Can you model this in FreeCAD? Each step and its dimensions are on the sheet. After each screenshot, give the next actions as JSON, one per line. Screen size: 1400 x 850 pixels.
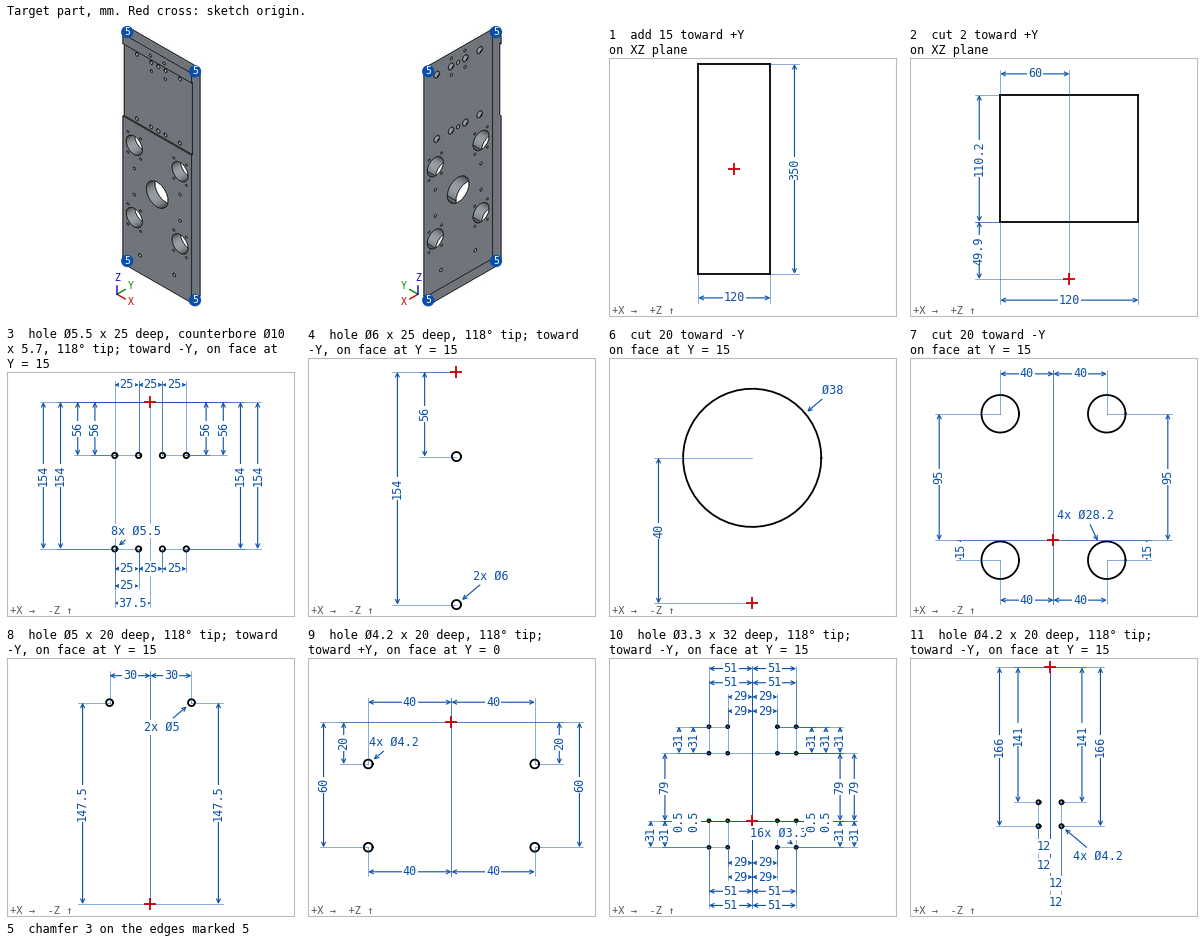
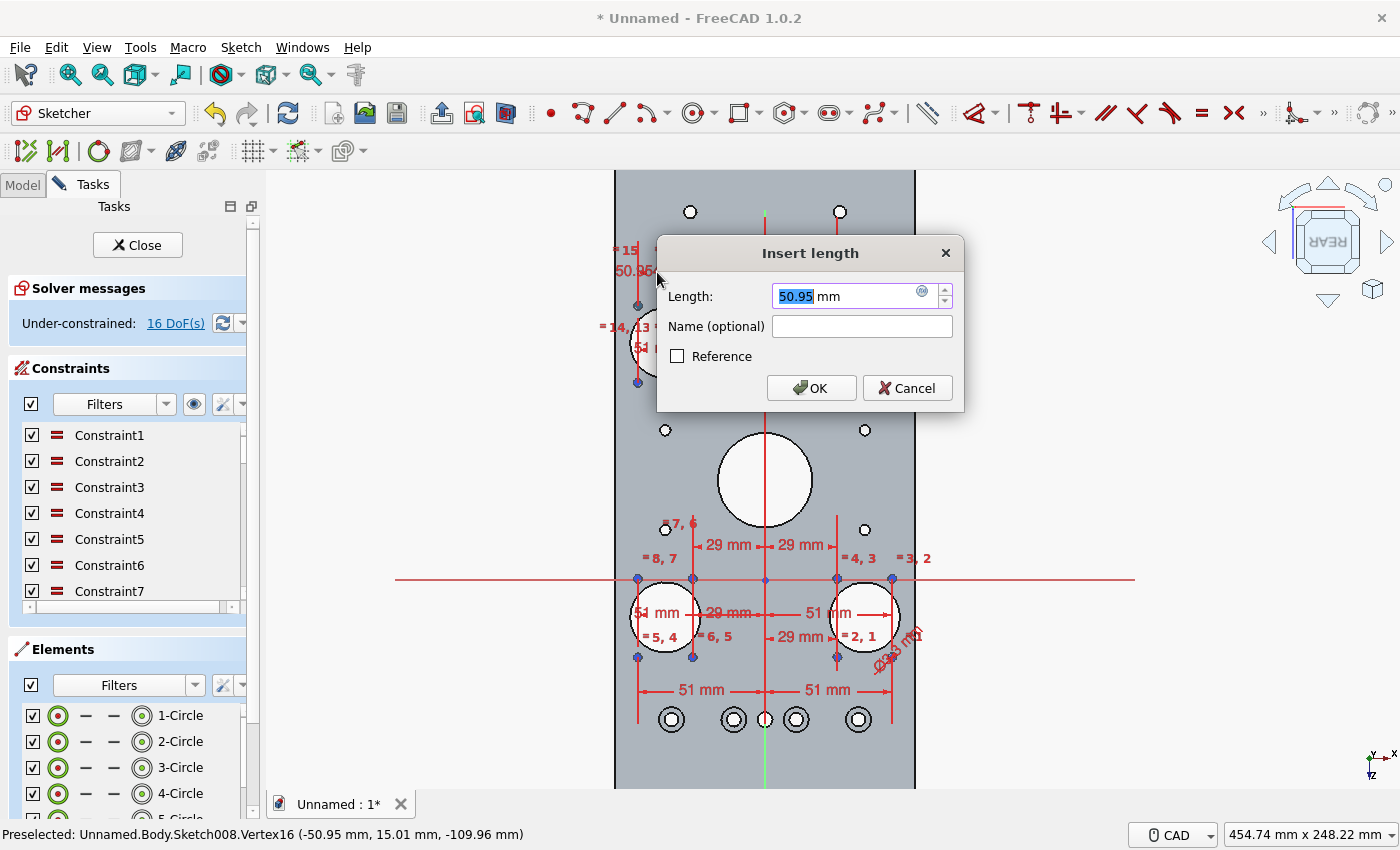
{"action": "type", "text": "51"}
{"action": "key", "text": "Return"}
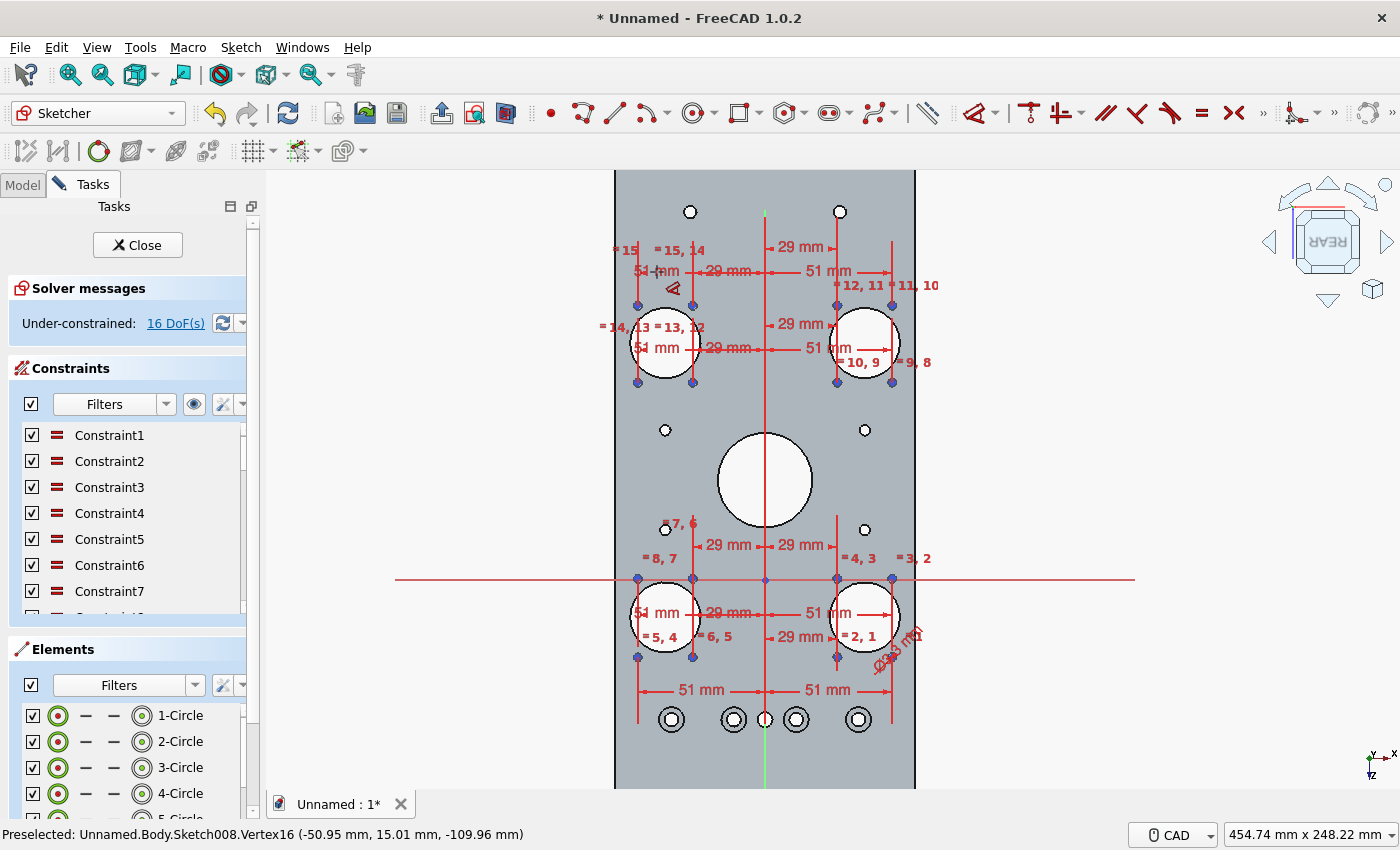
{"action": "scroll", "coordinate": [892, 579], "scroll_direction": "up", "scroll_amount": 18}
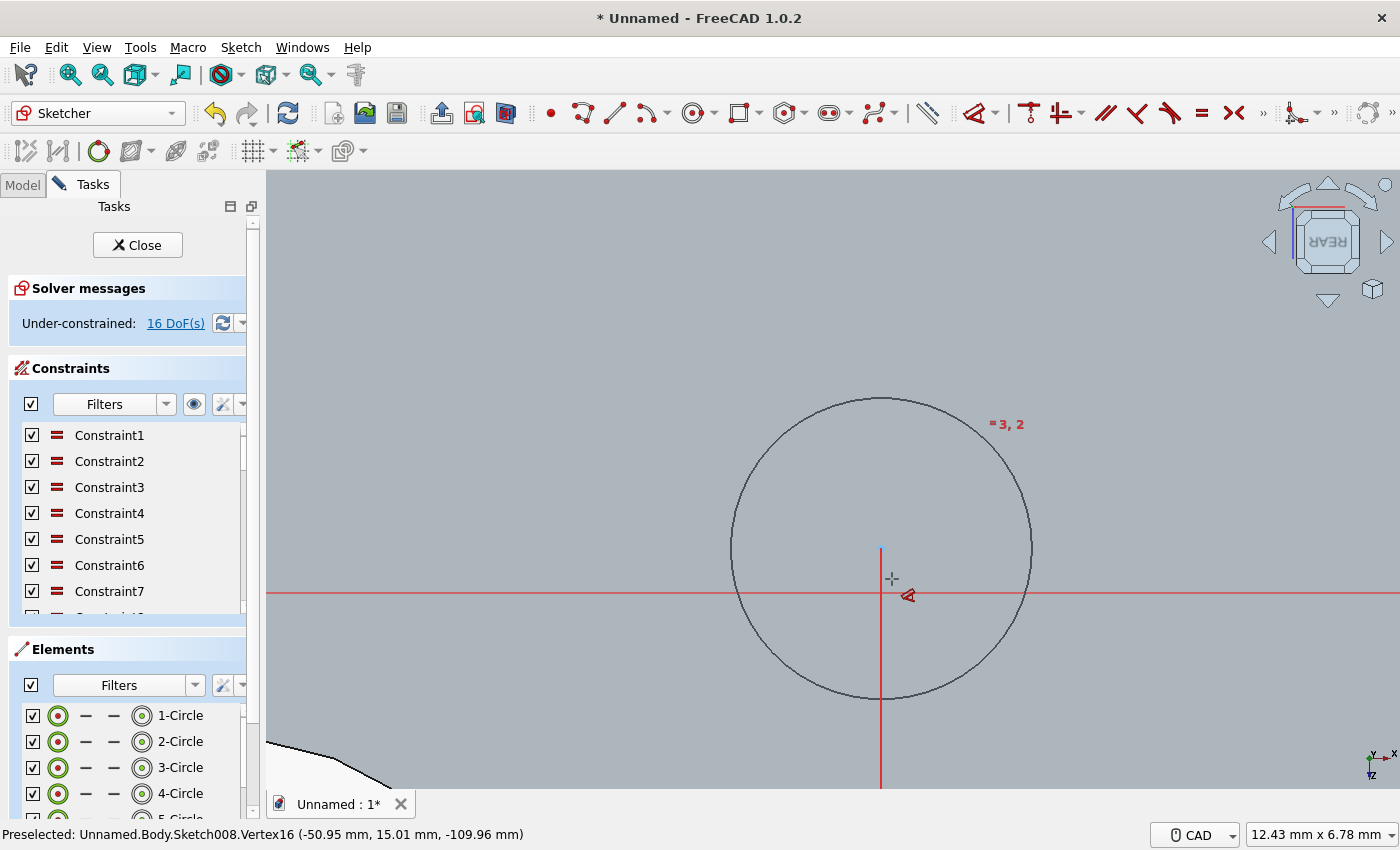
{"action": "left_click", "coordinate": [881, 549]}
{"action": "left_click", "coordinate": [915, 571]}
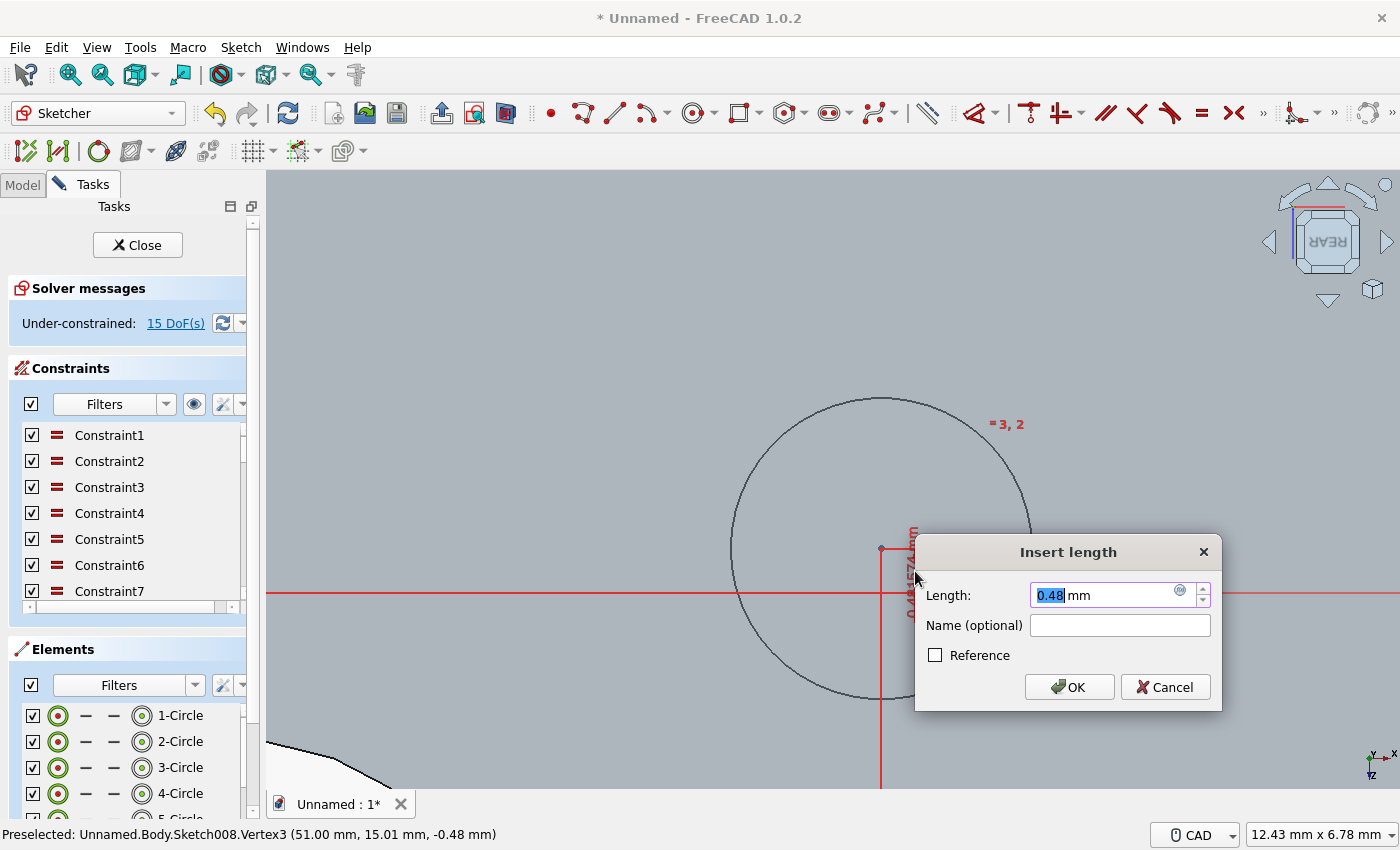
{"action": "type", "text": "0.5"}
{"action": "key", "text": "Return"}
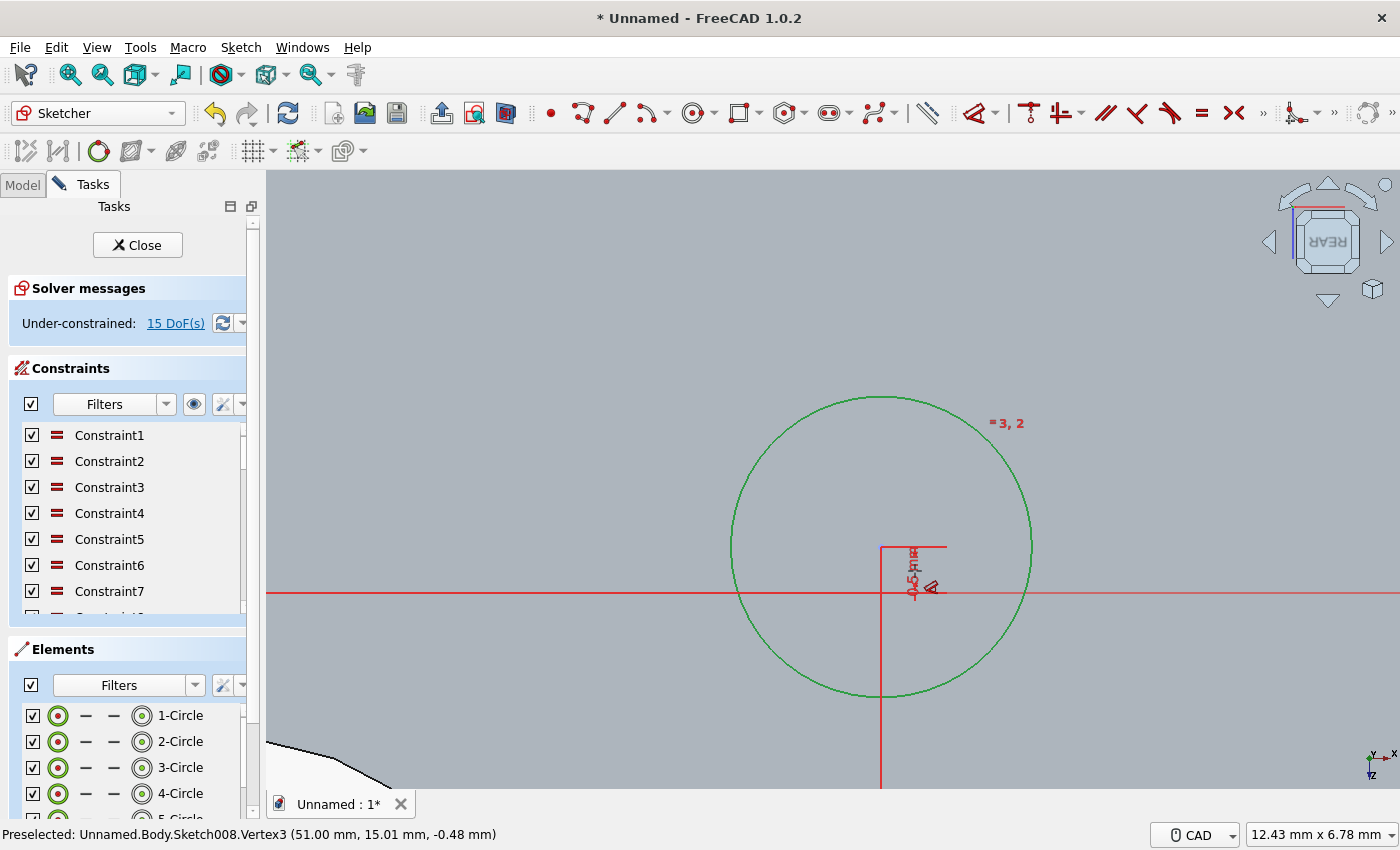
{"action": "scroll", "coordinate": [921, 602], "scroll_direction": "down", "scroll_amount": 17}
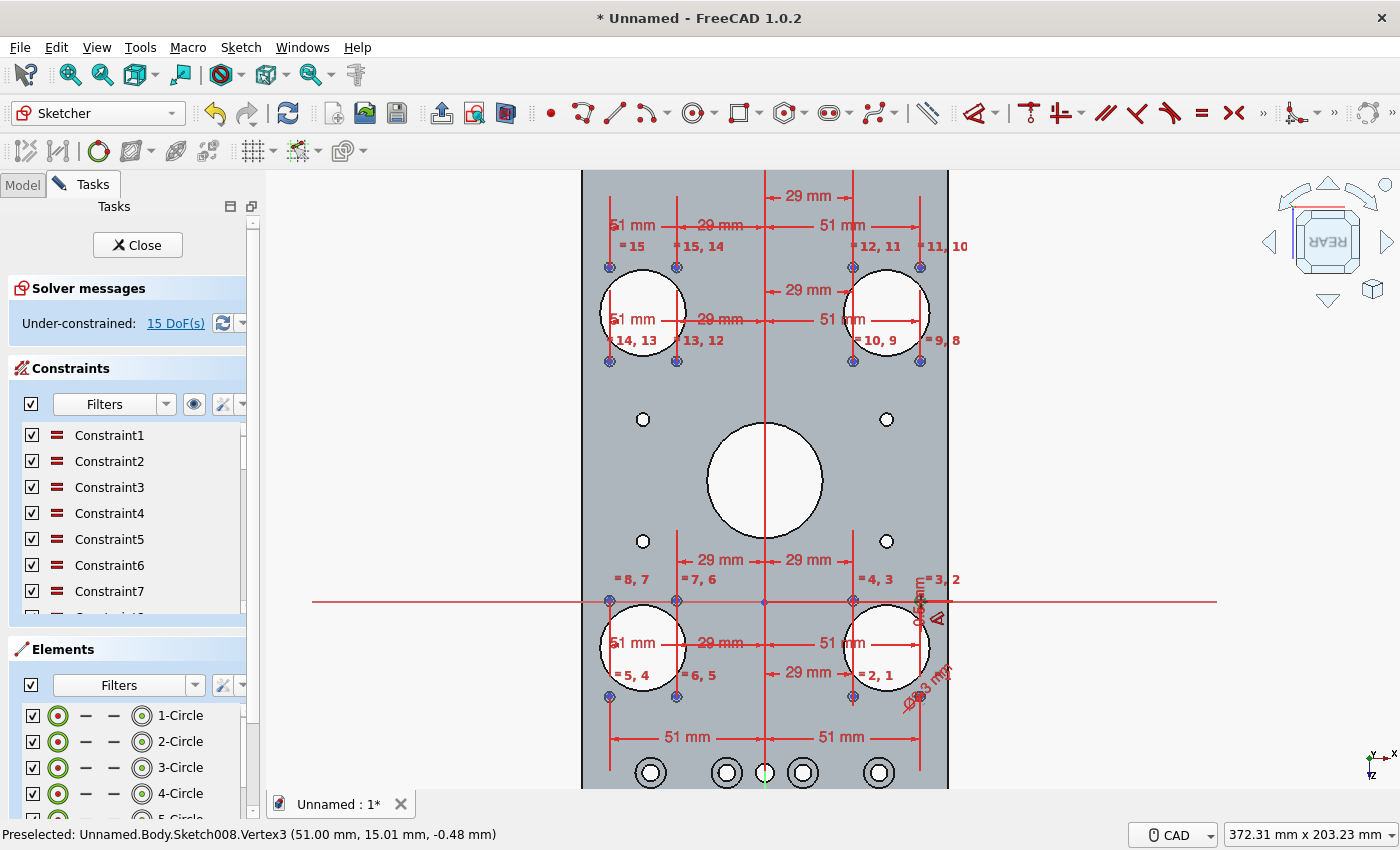
{"action": "scroll", "coordinate": [853, 601], "scroll_direction": "up", "scroll_amount": 17}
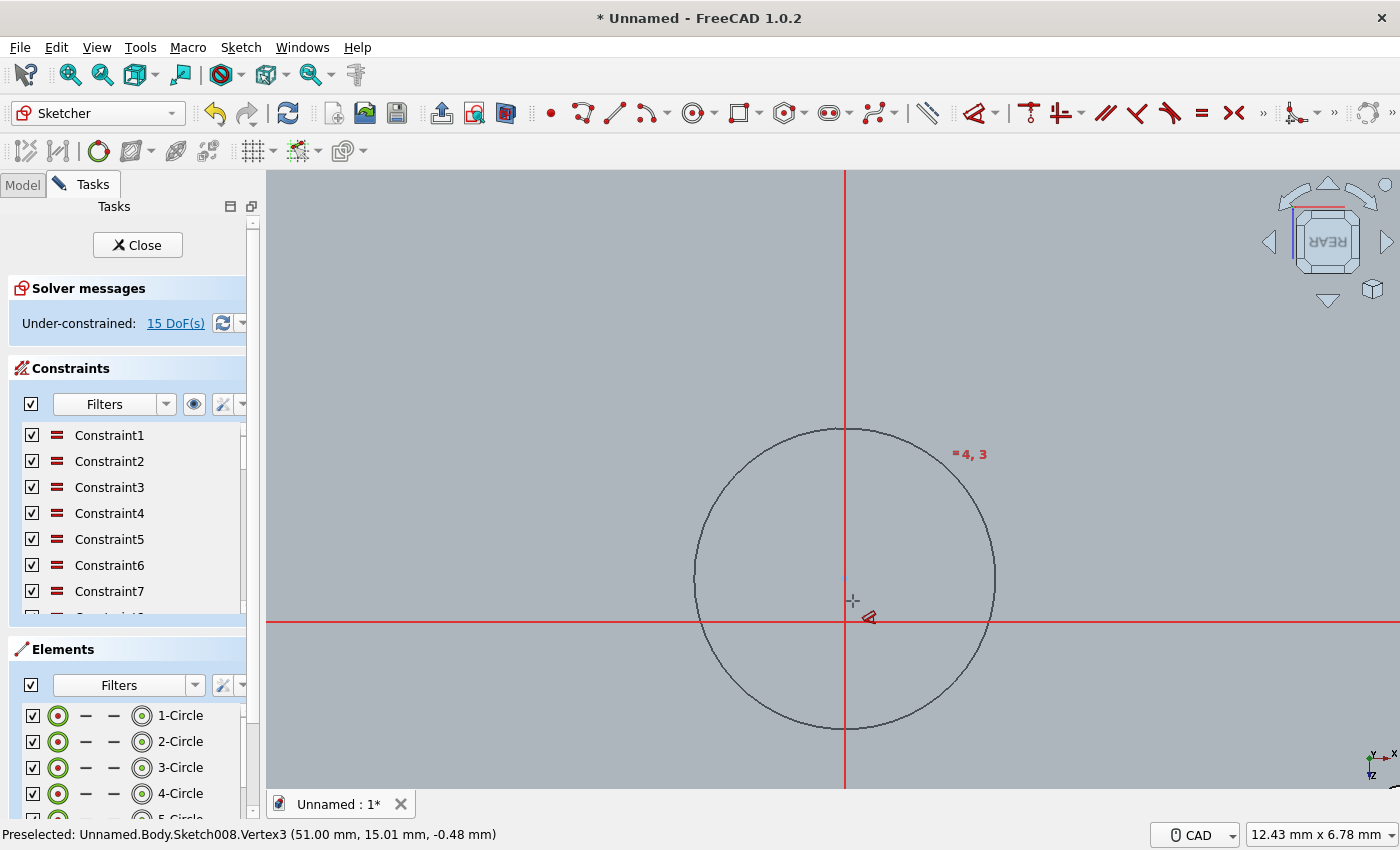
{"action": "left_click", "coordinate": [845, 579]}
{"action": "left_click", "coordinate": [879, 600]}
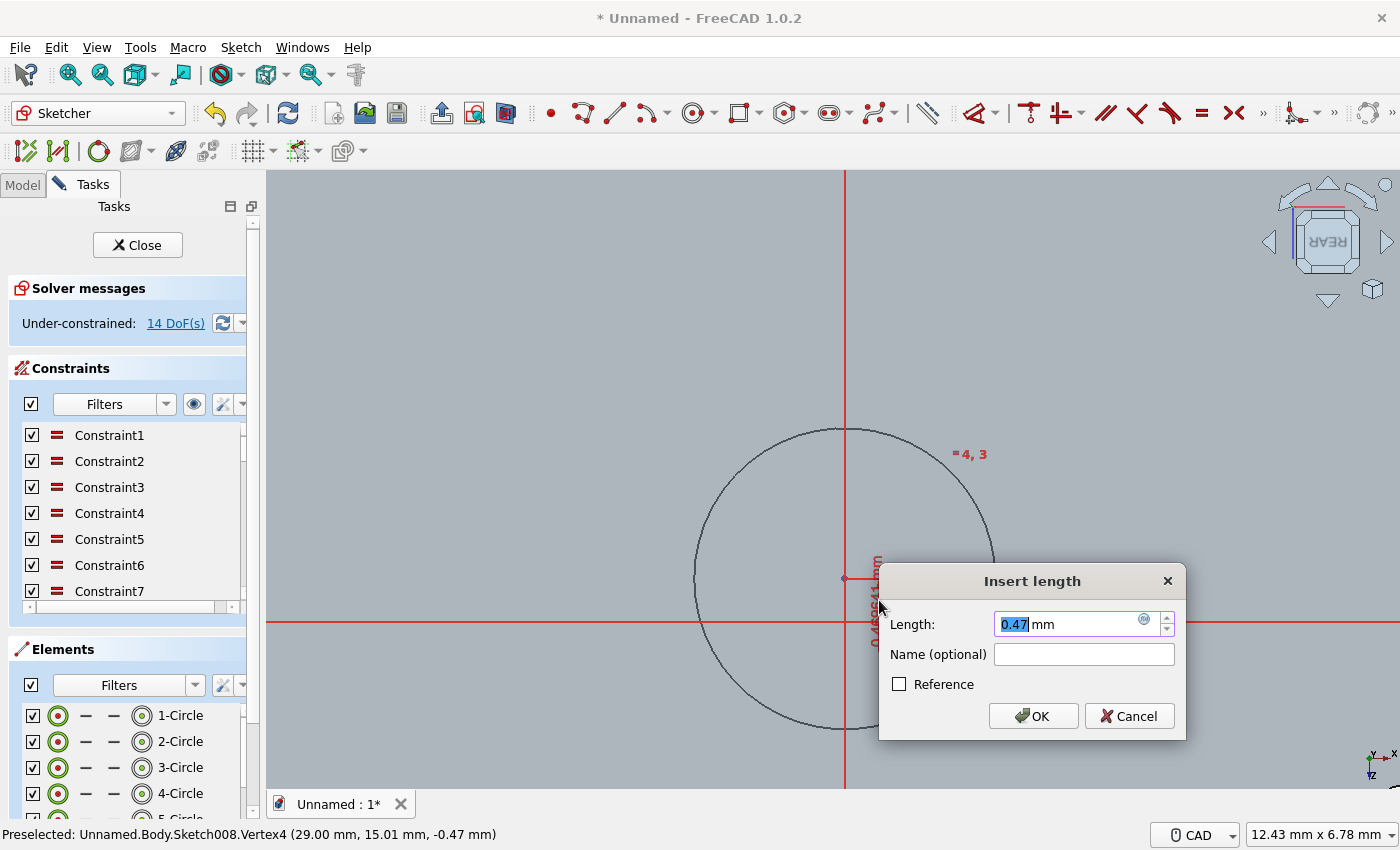
{"action": "type", "text": "0.5"}
{"action": "key", "text": "Return"}